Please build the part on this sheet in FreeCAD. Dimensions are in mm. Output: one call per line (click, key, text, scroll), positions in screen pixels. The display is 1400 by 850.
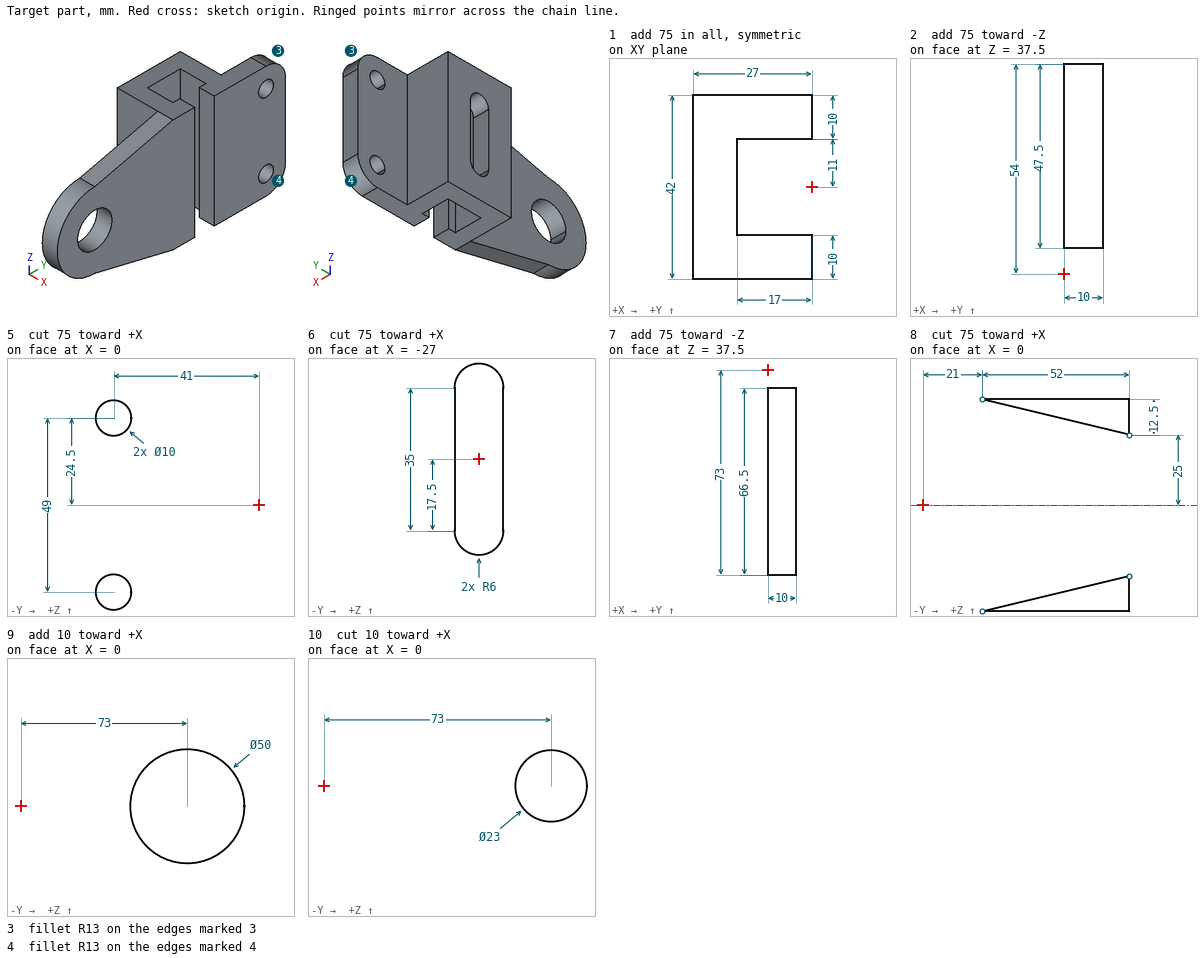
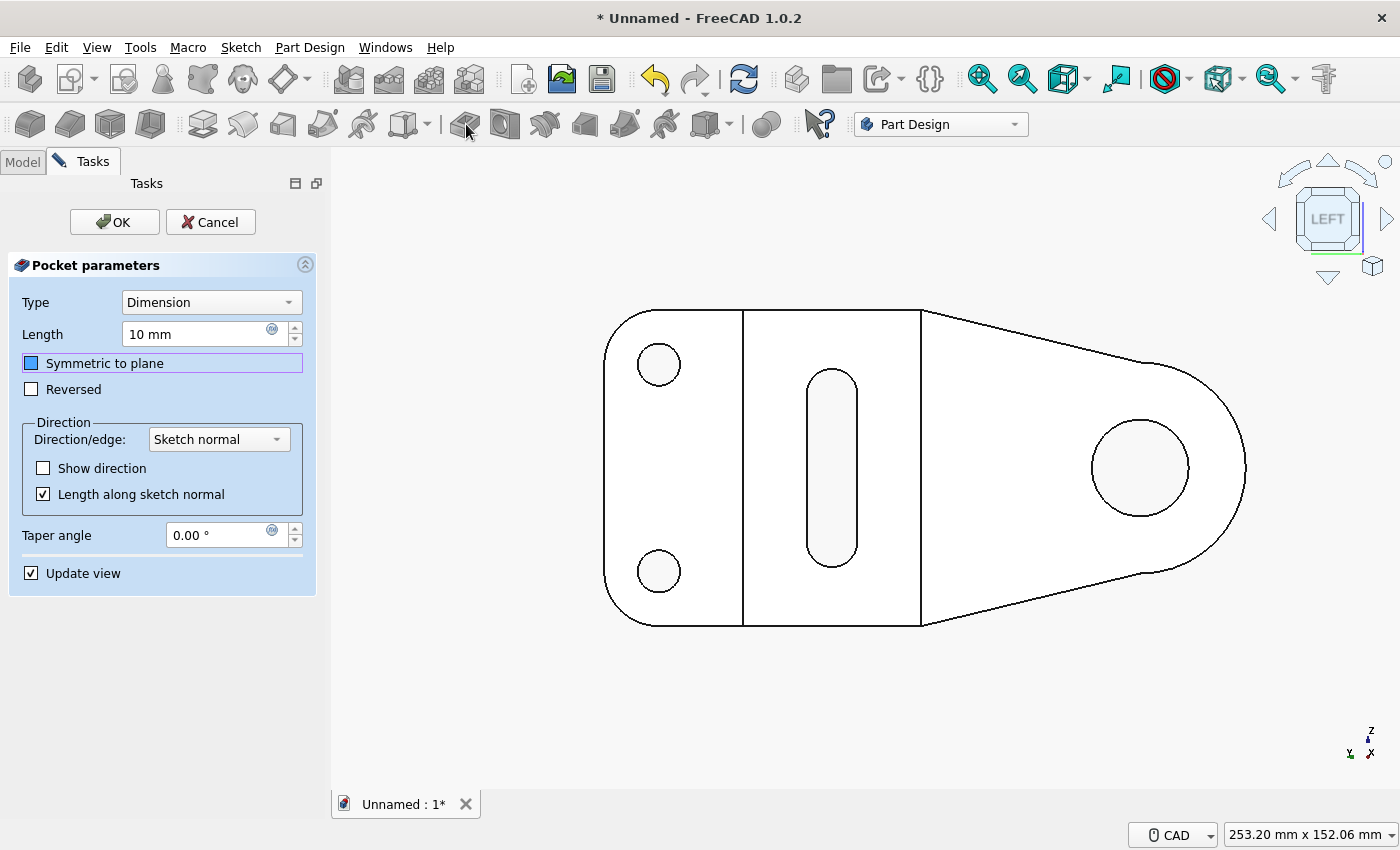
click(115, 222)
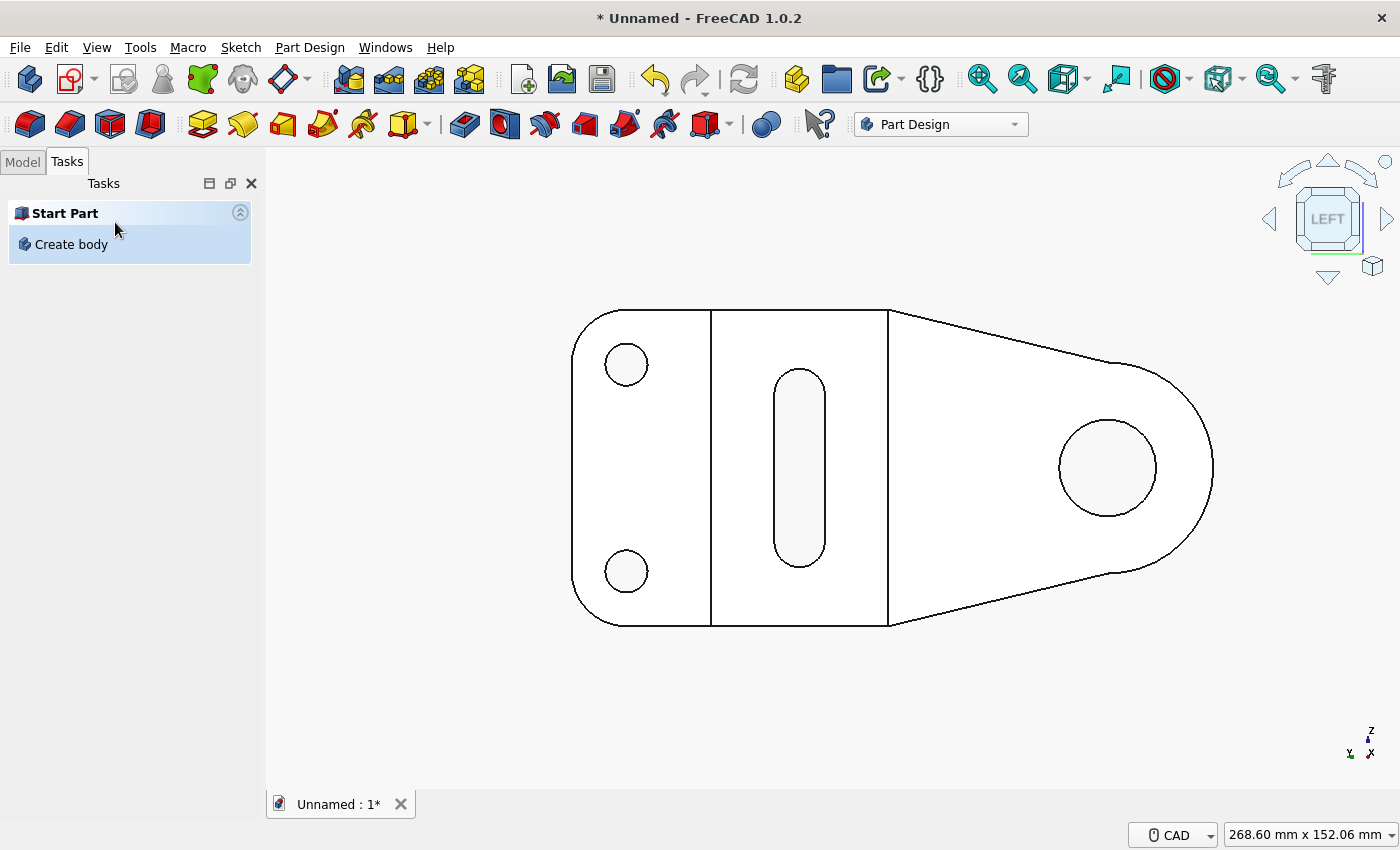
key(0)